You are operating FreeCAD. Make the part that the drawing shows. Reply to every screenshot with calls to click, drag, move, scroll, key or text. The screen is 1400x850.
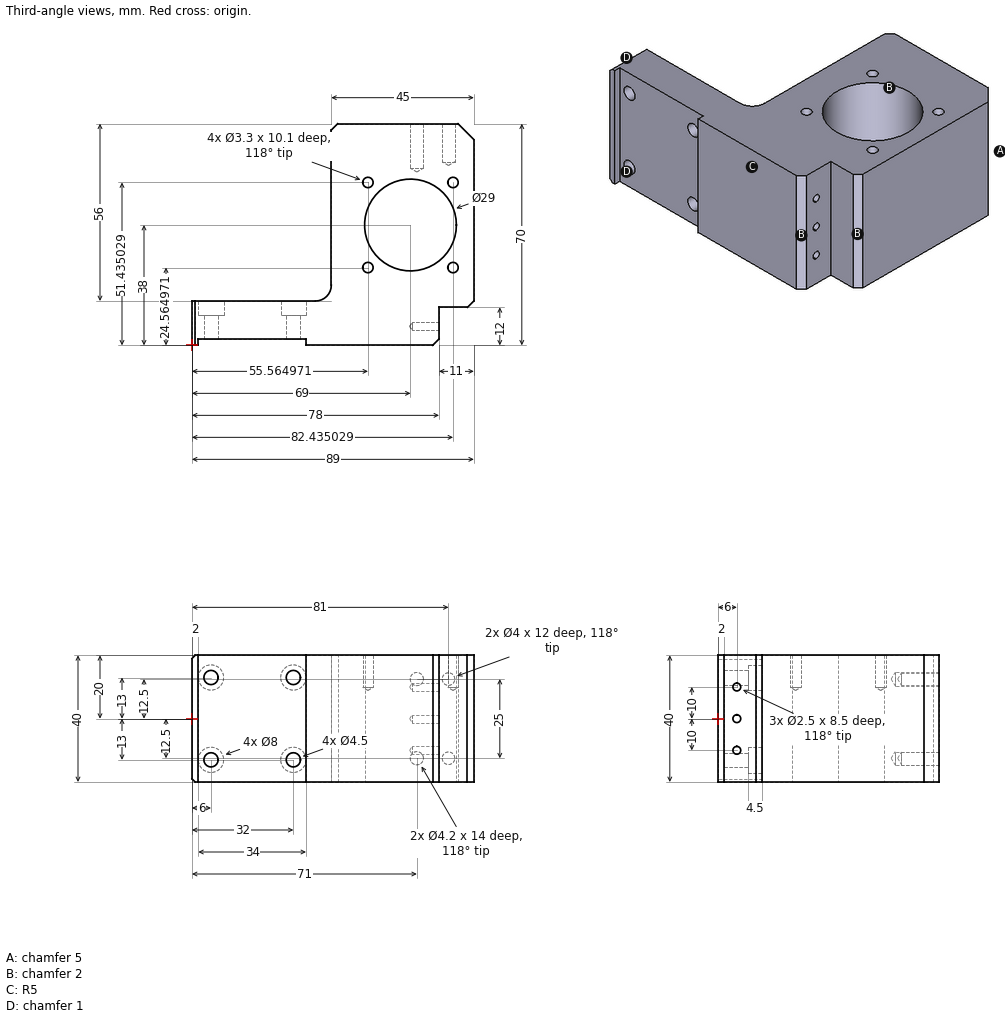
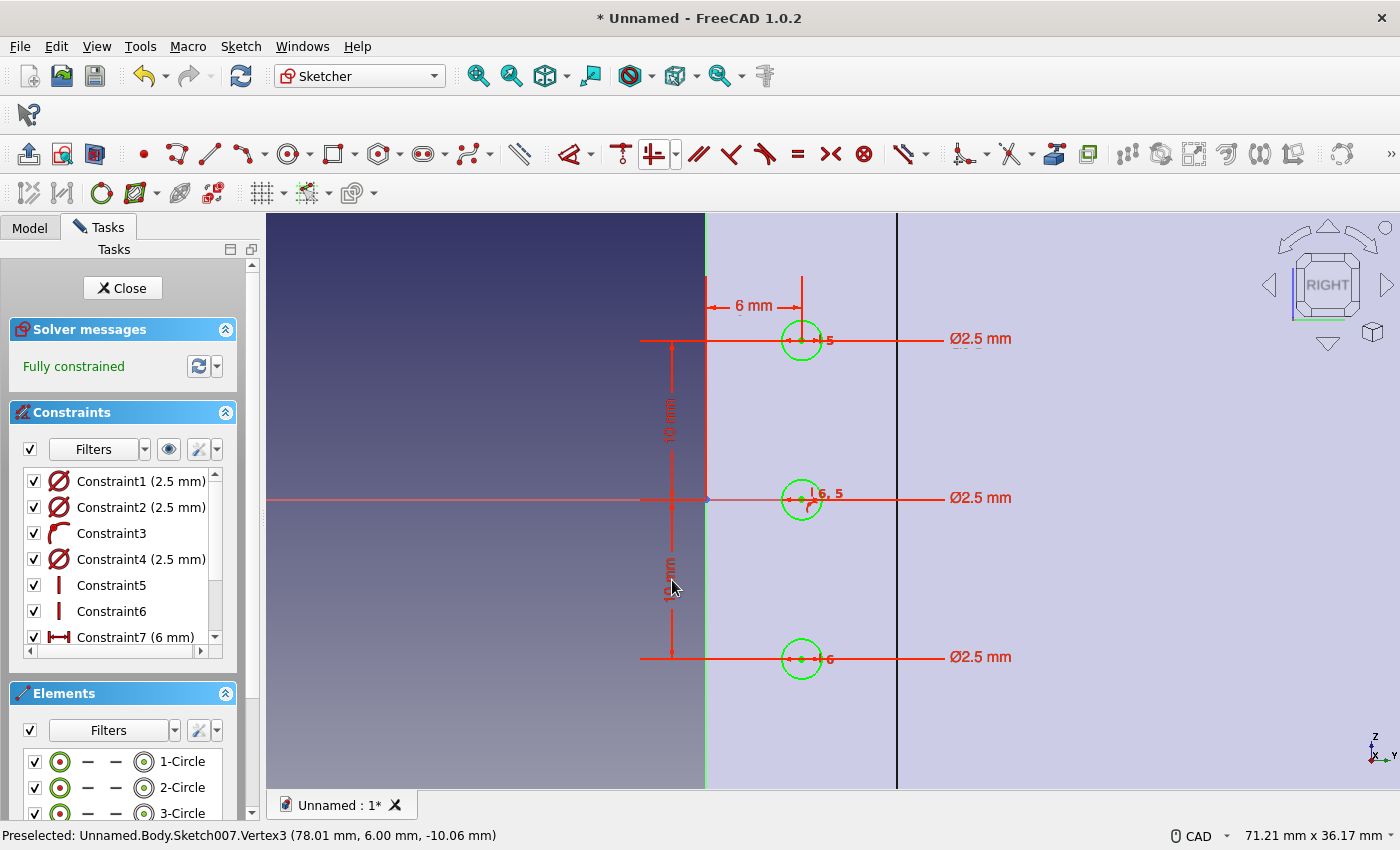
click(123, 288)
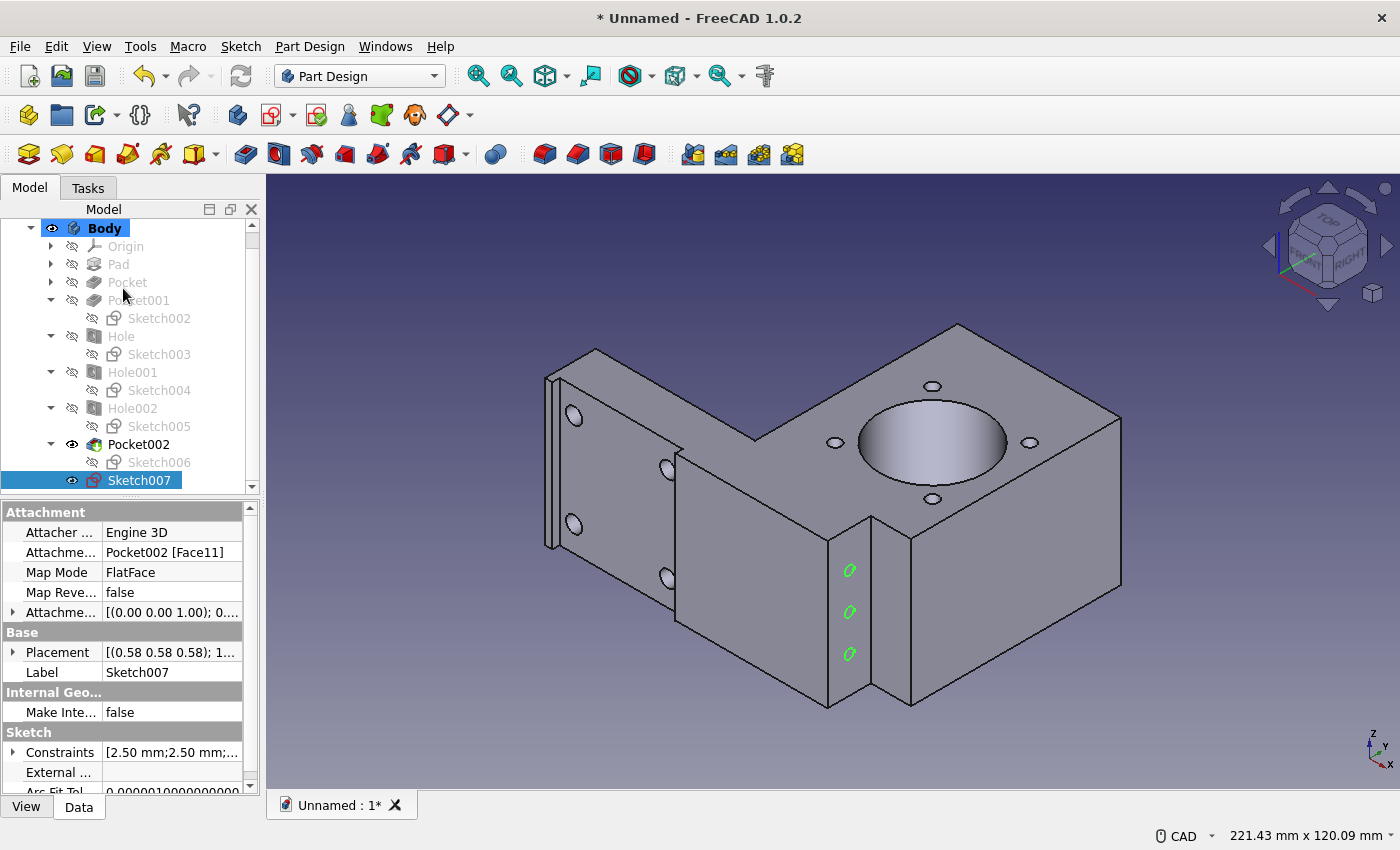
click(279, 154)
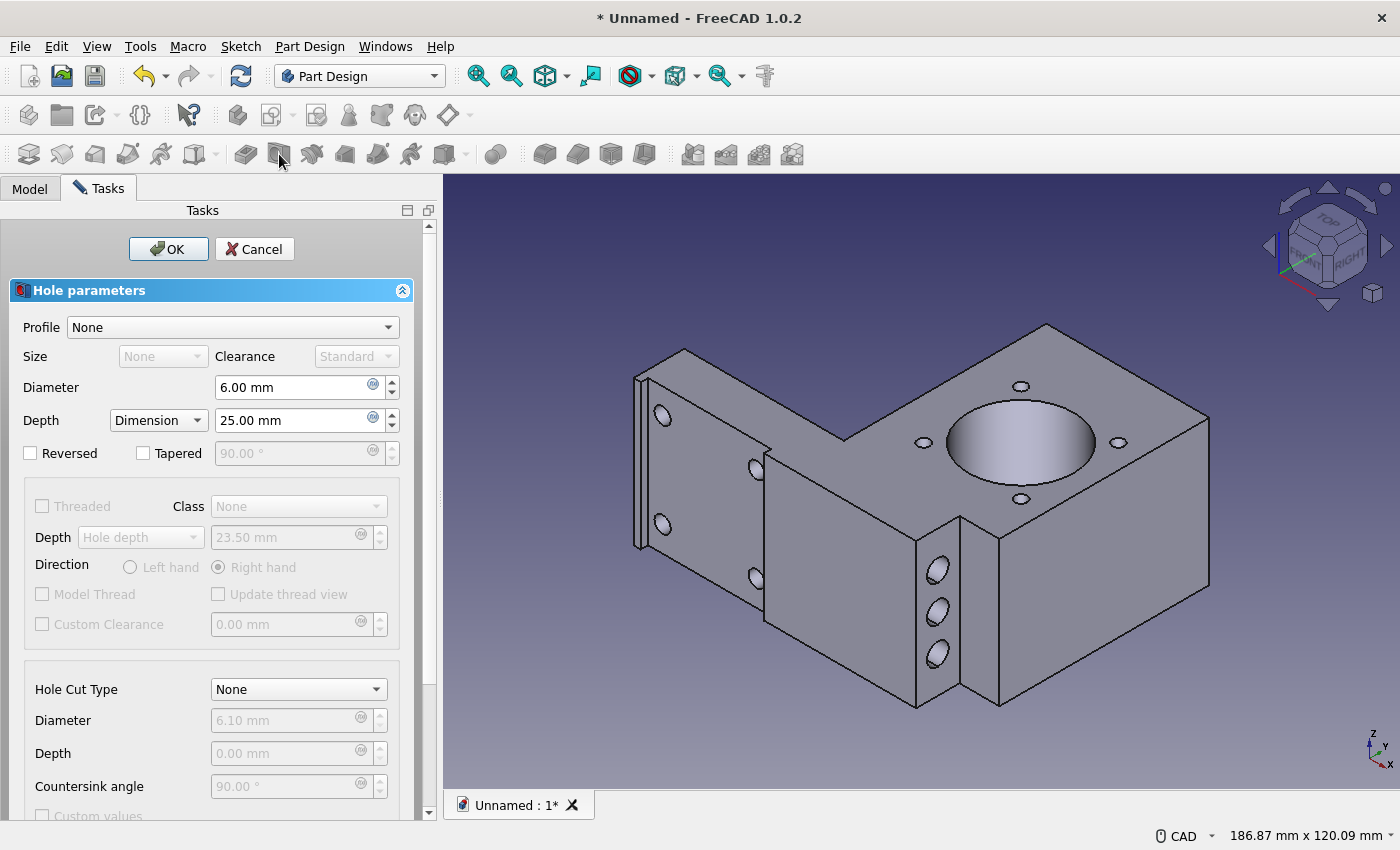
triple_click(300, 388)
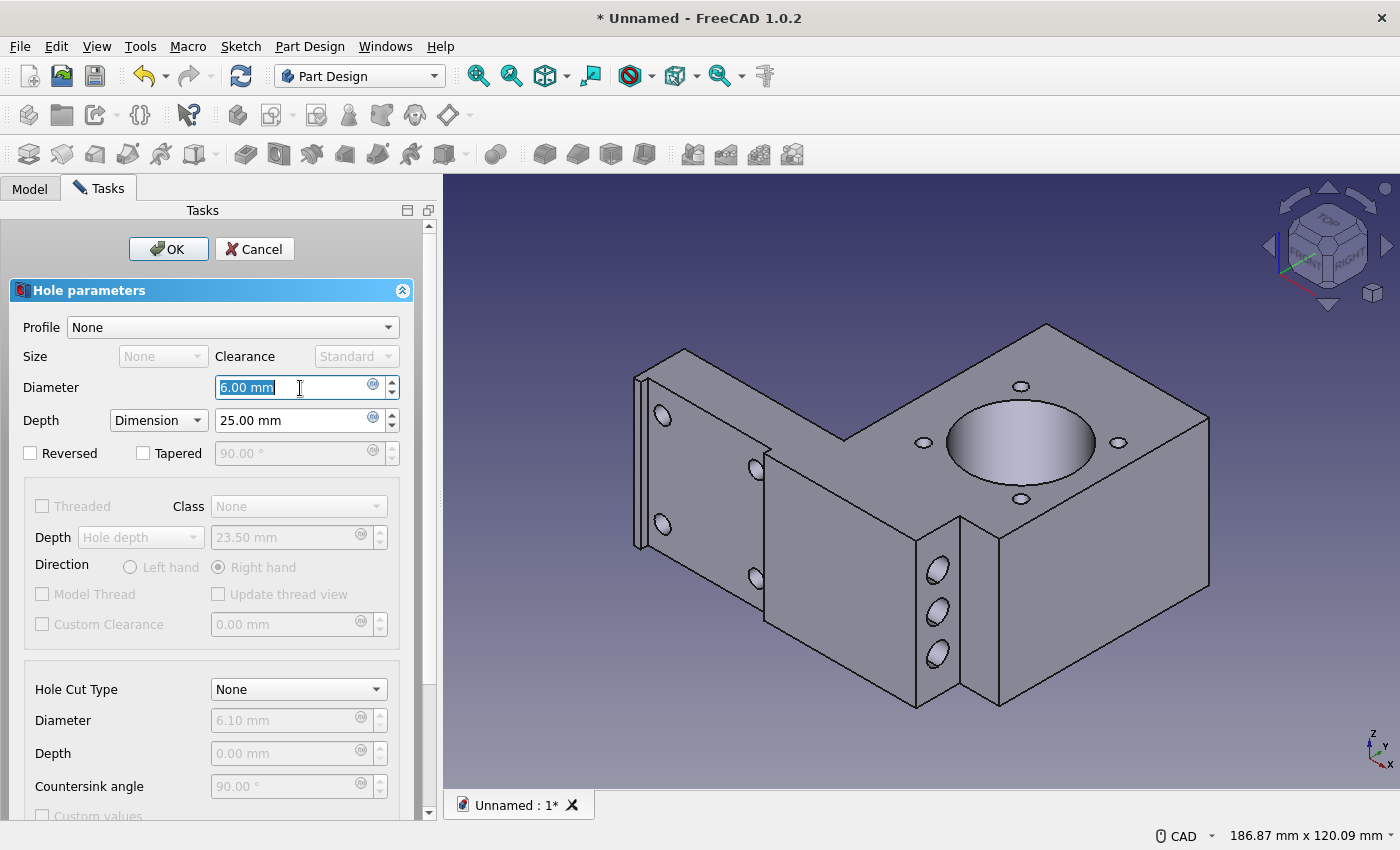
text(2.5)
key(Tab)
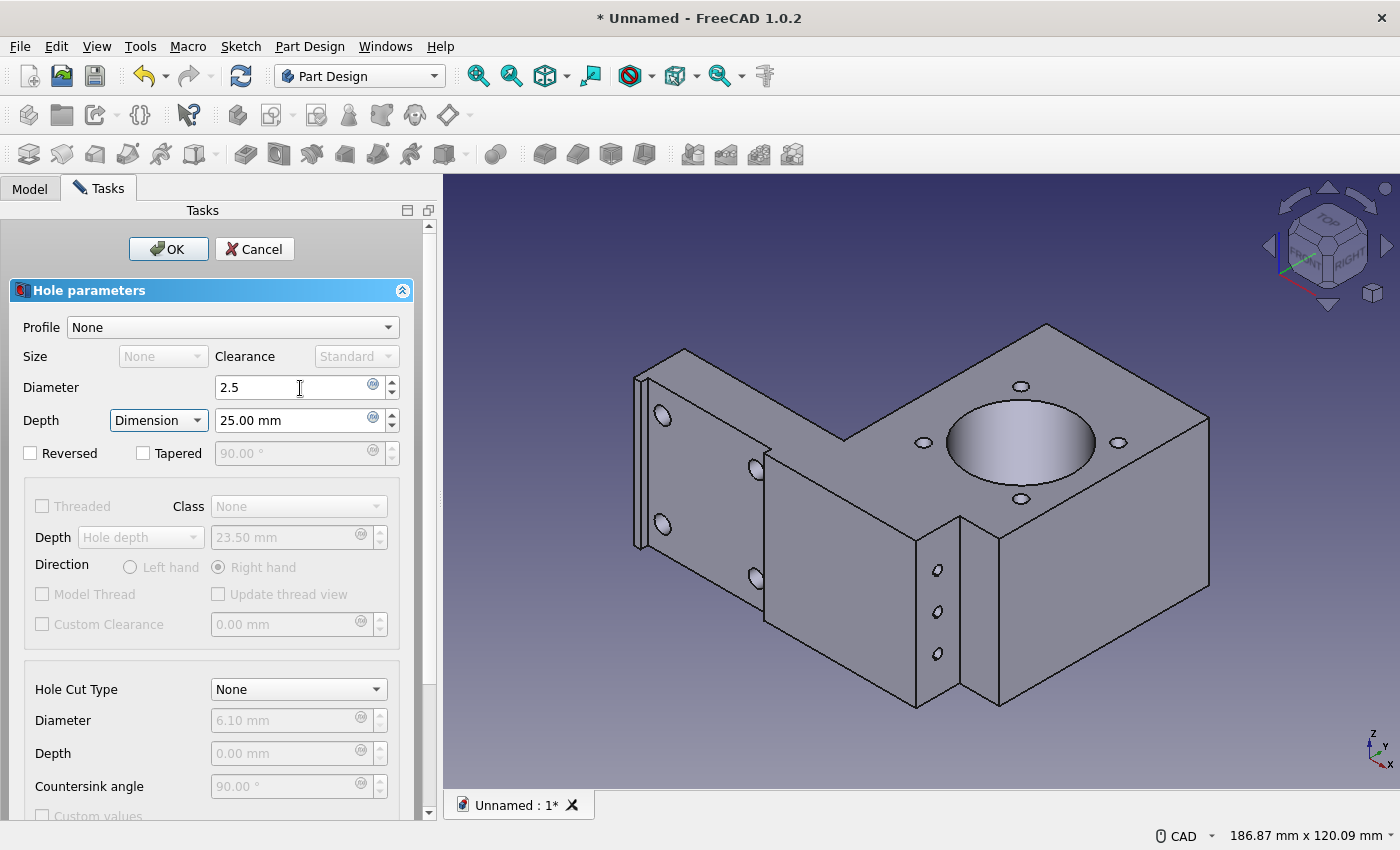
triple_click(300, 420)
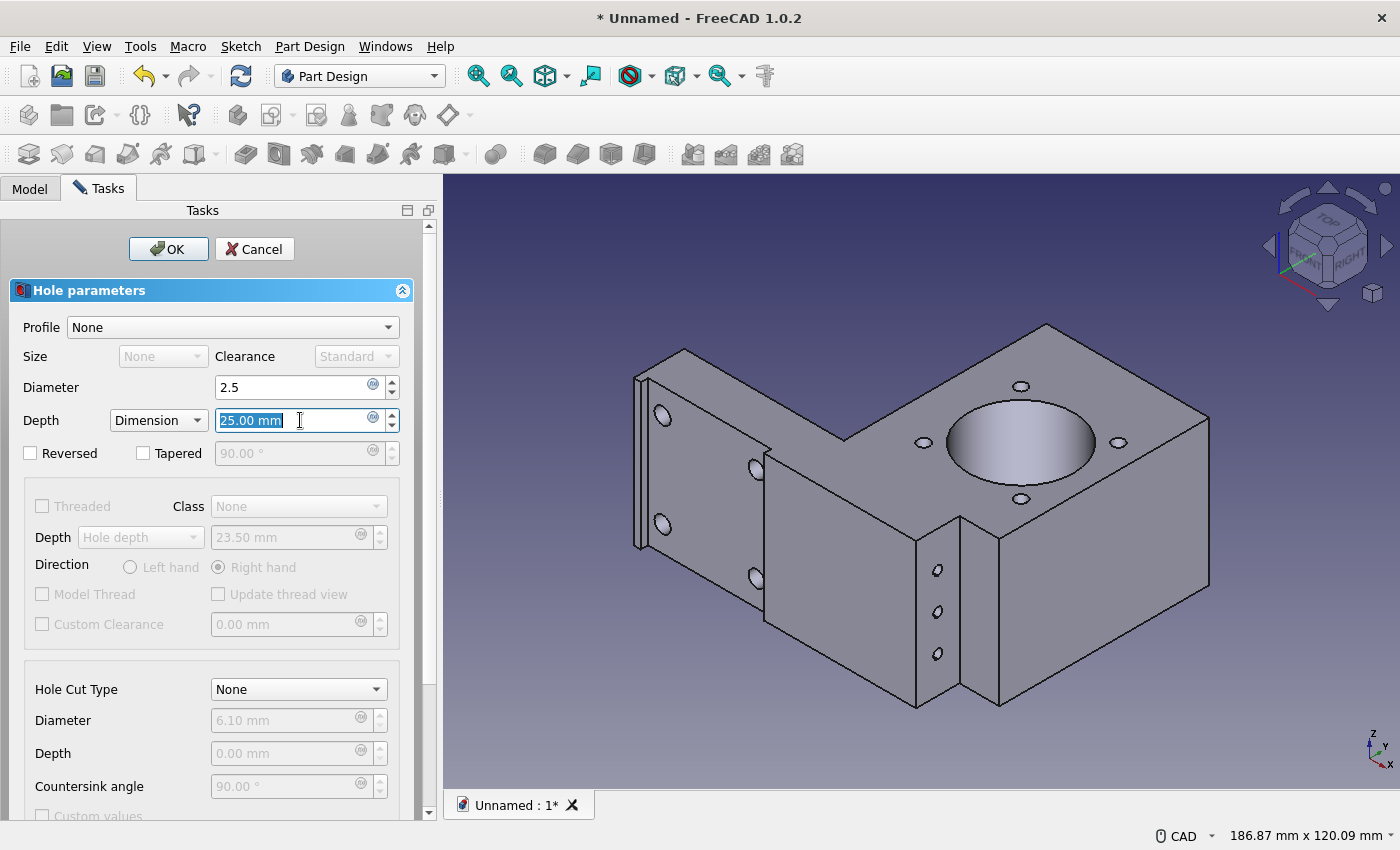
text(8.5)
key(Tab)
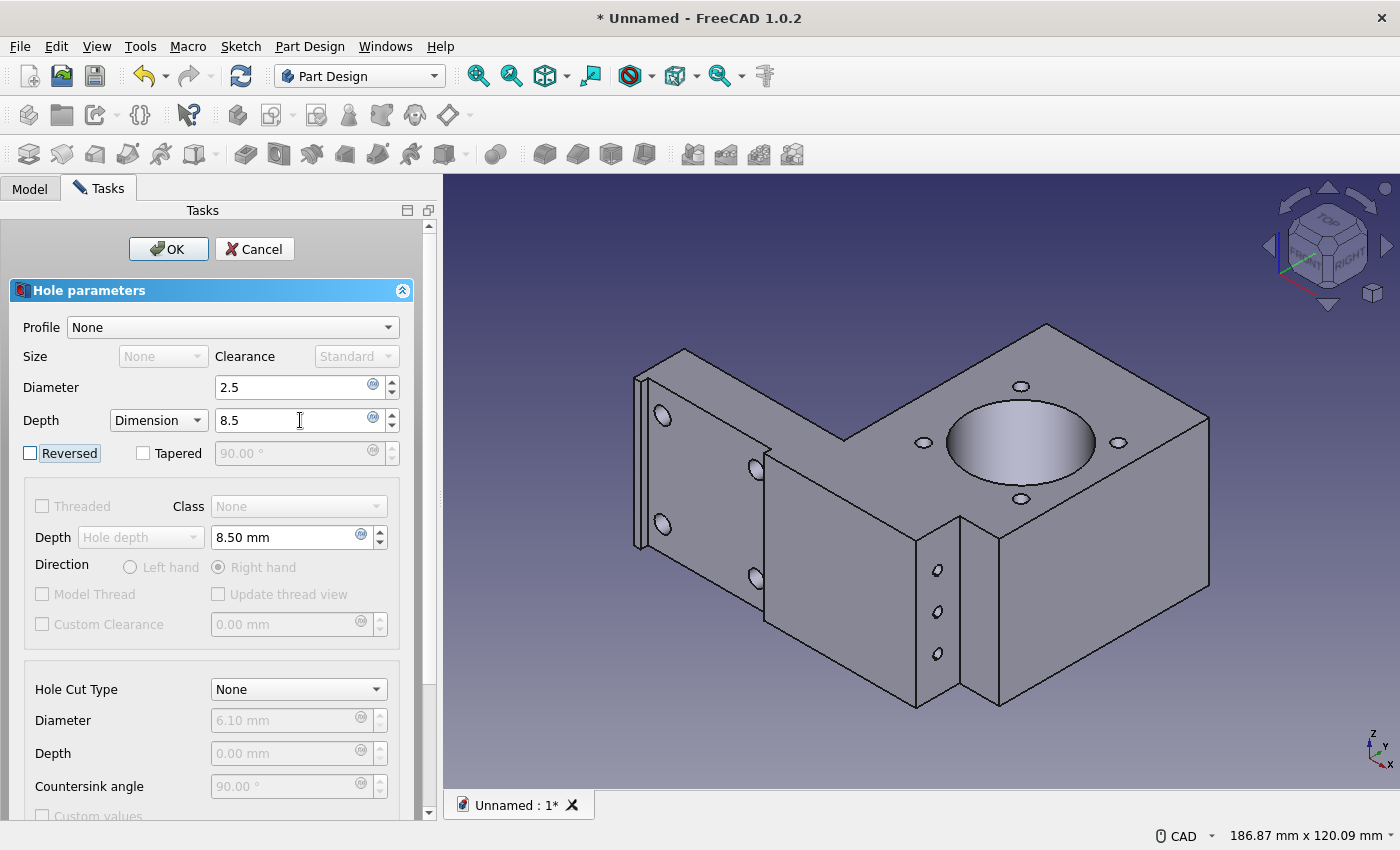
click(169, 249)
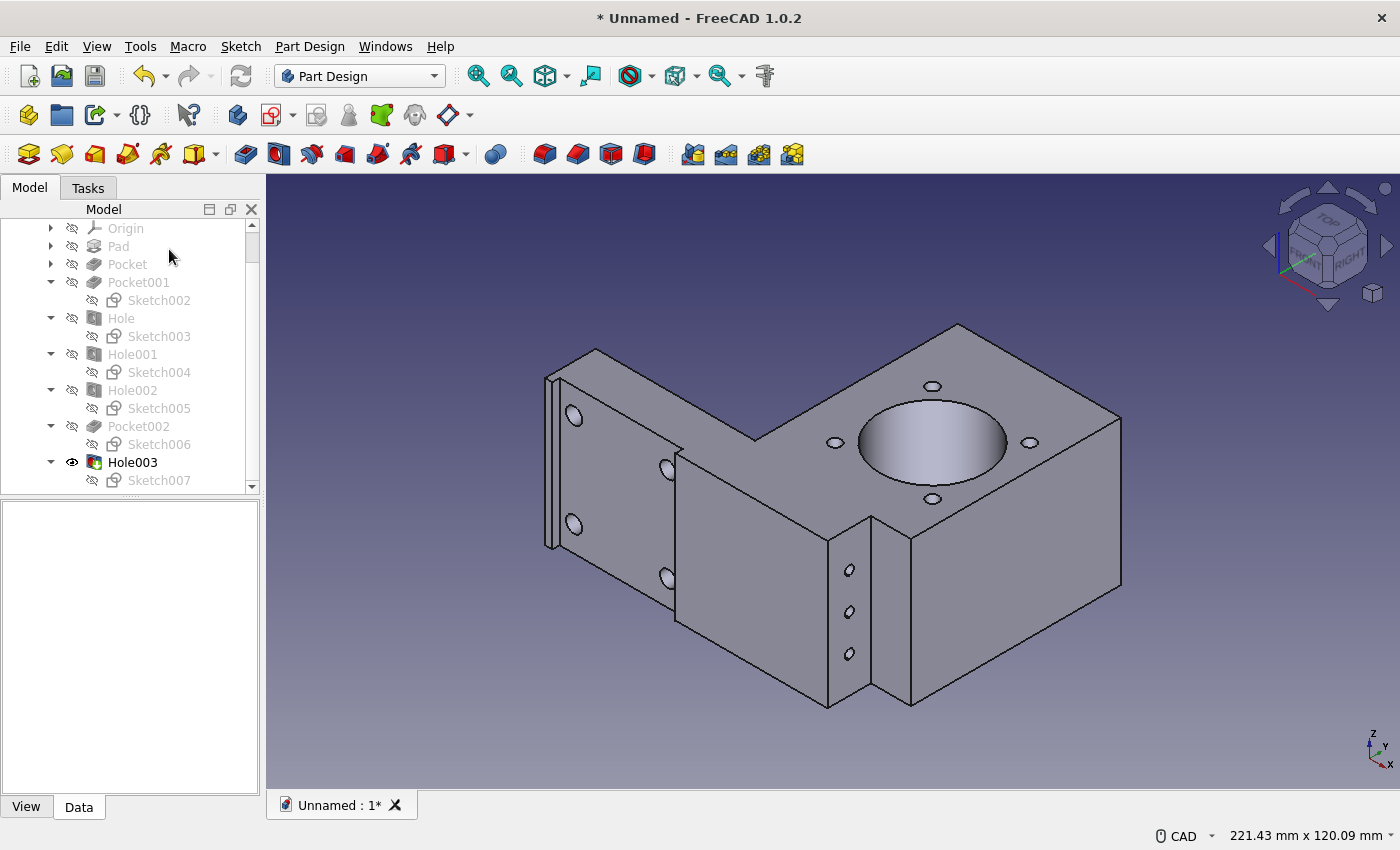
key(2)